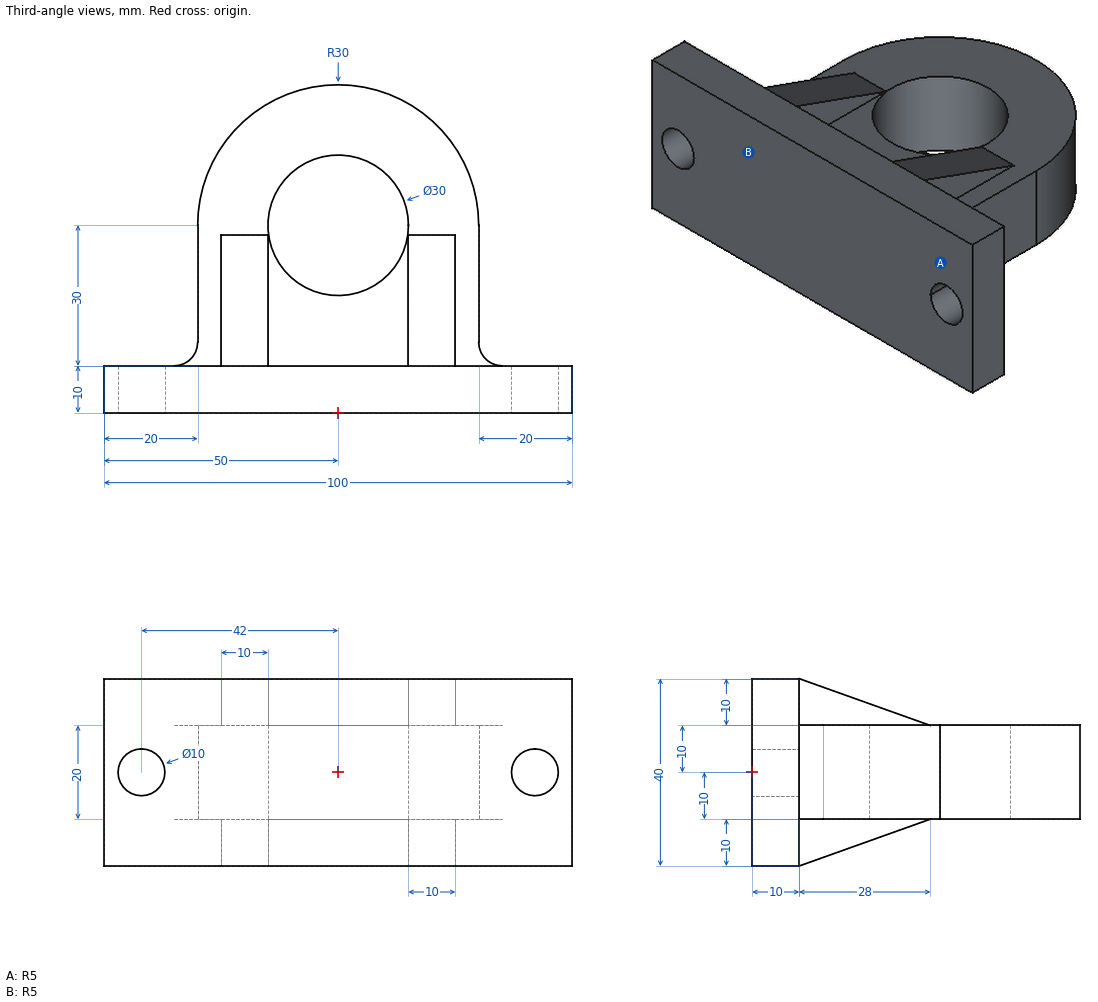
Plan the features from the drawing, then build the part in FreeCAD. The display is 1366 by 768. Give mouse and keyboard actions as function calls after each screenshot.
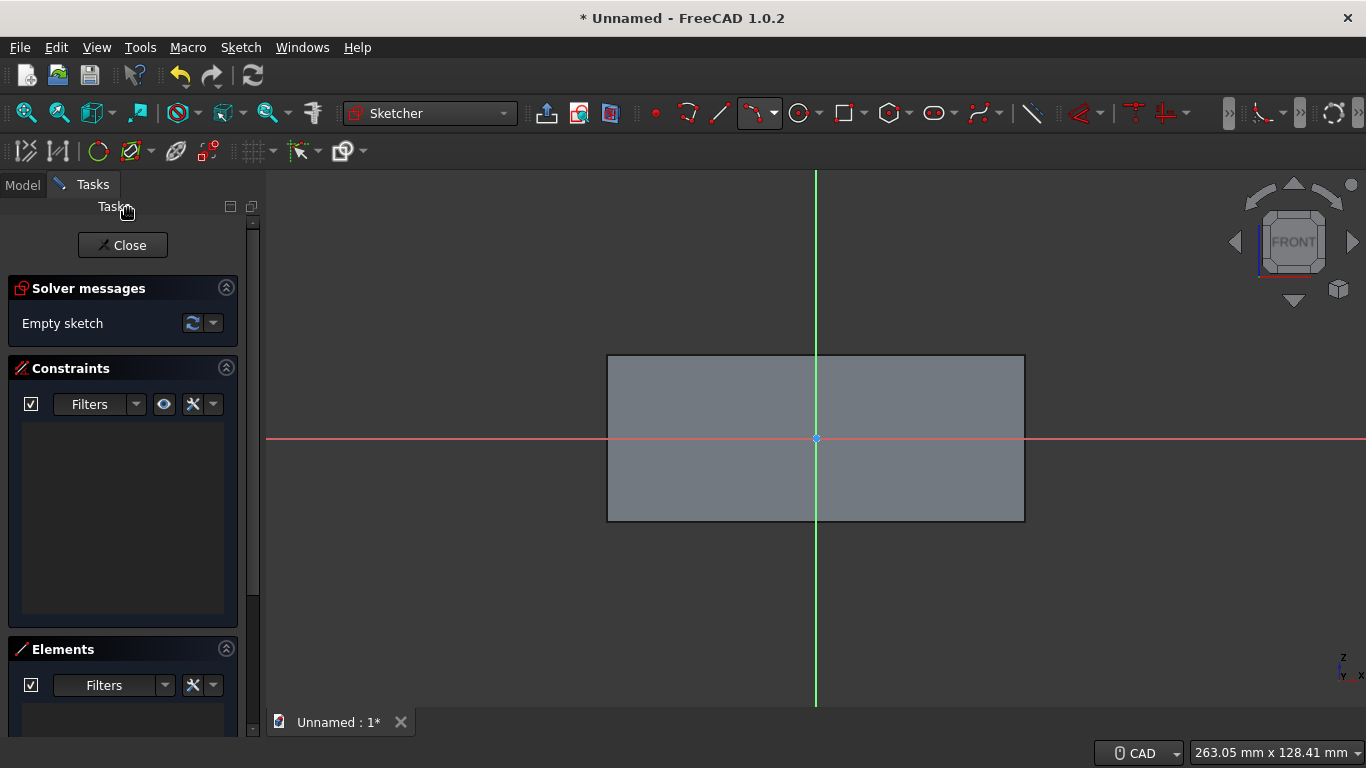
scroll(624, 438, up, 10)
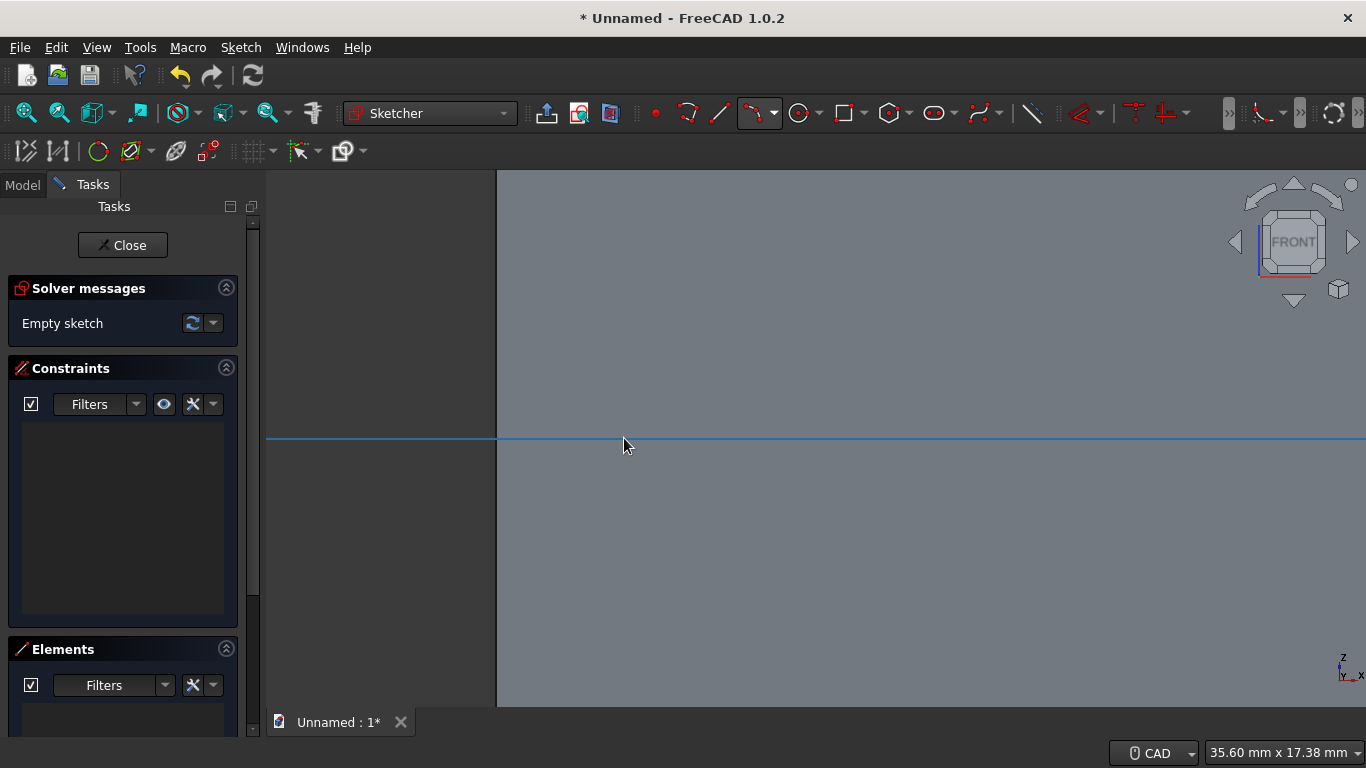
click(800, 114)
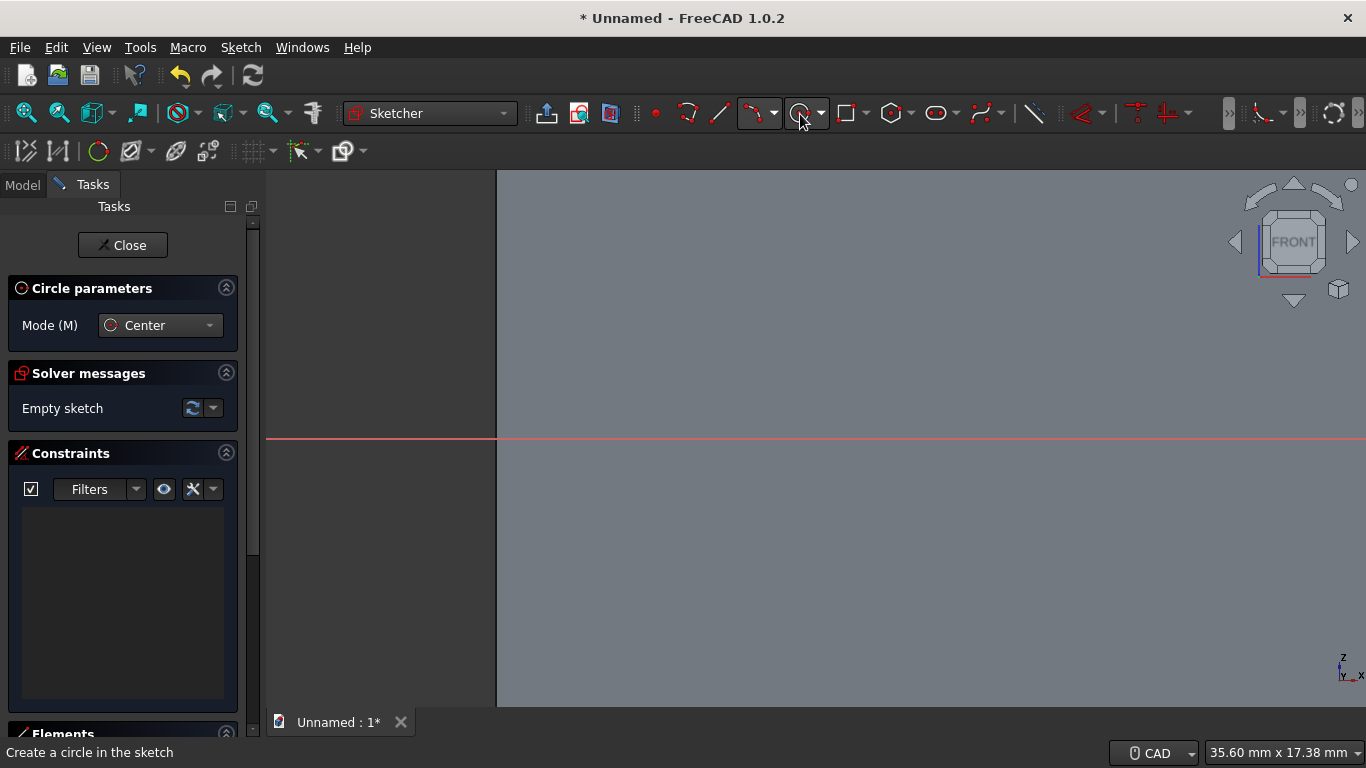
click(743, 438)
move(852, 329)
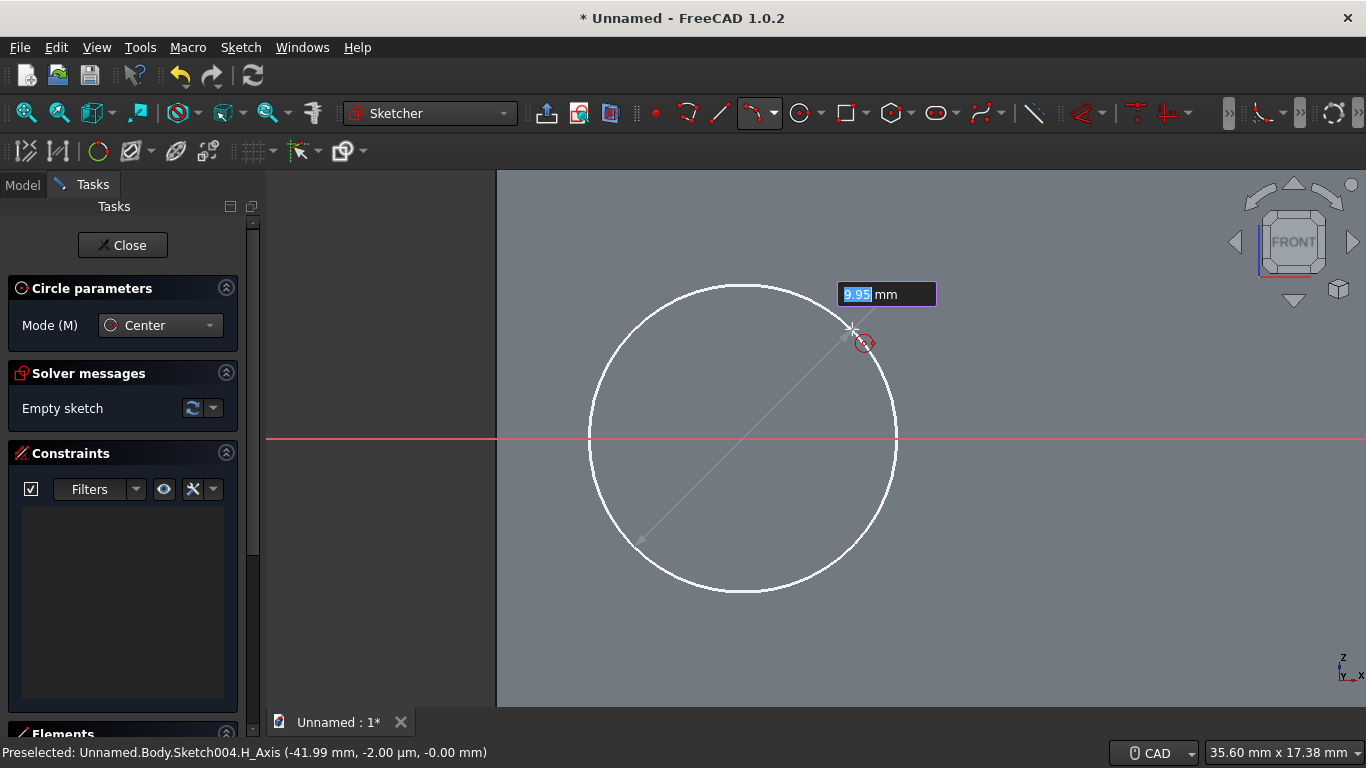
text(10)
key(Return)
key(Escape)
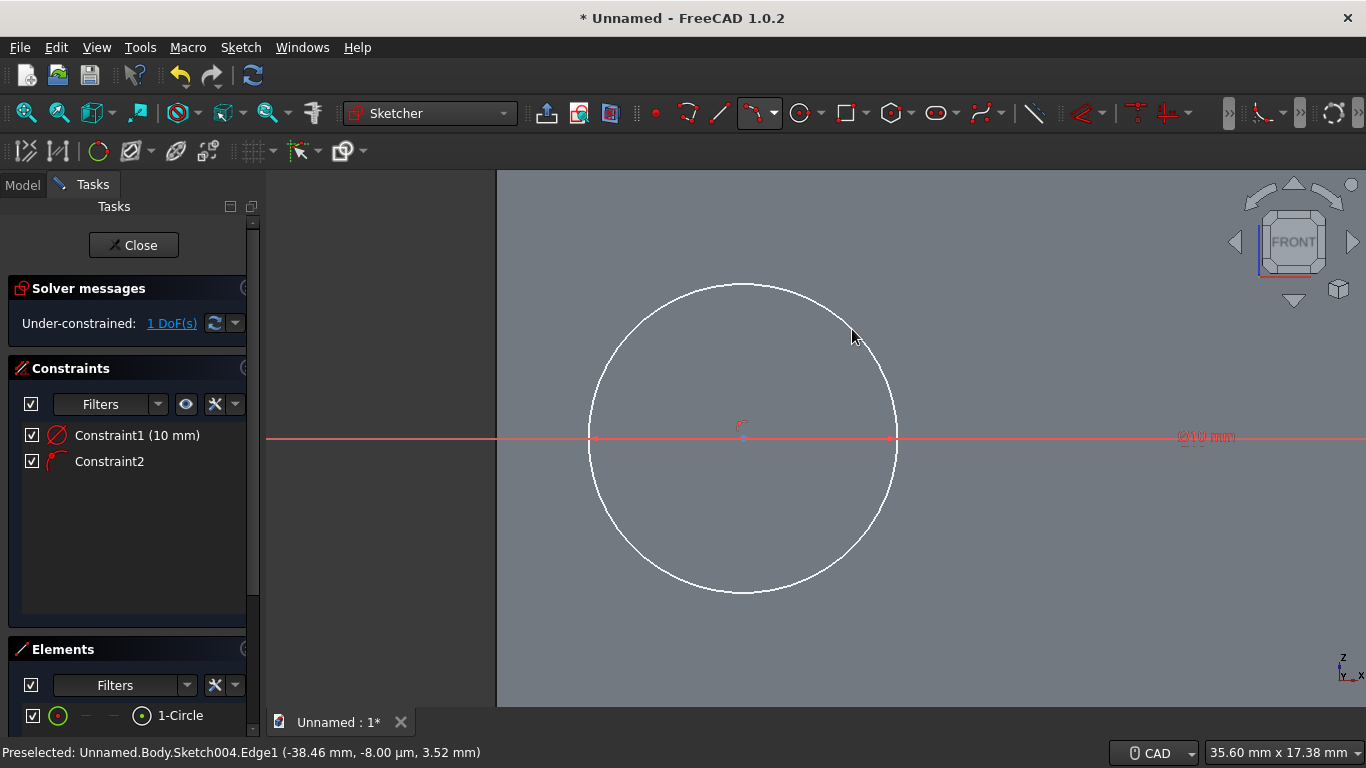
click(1082, 114)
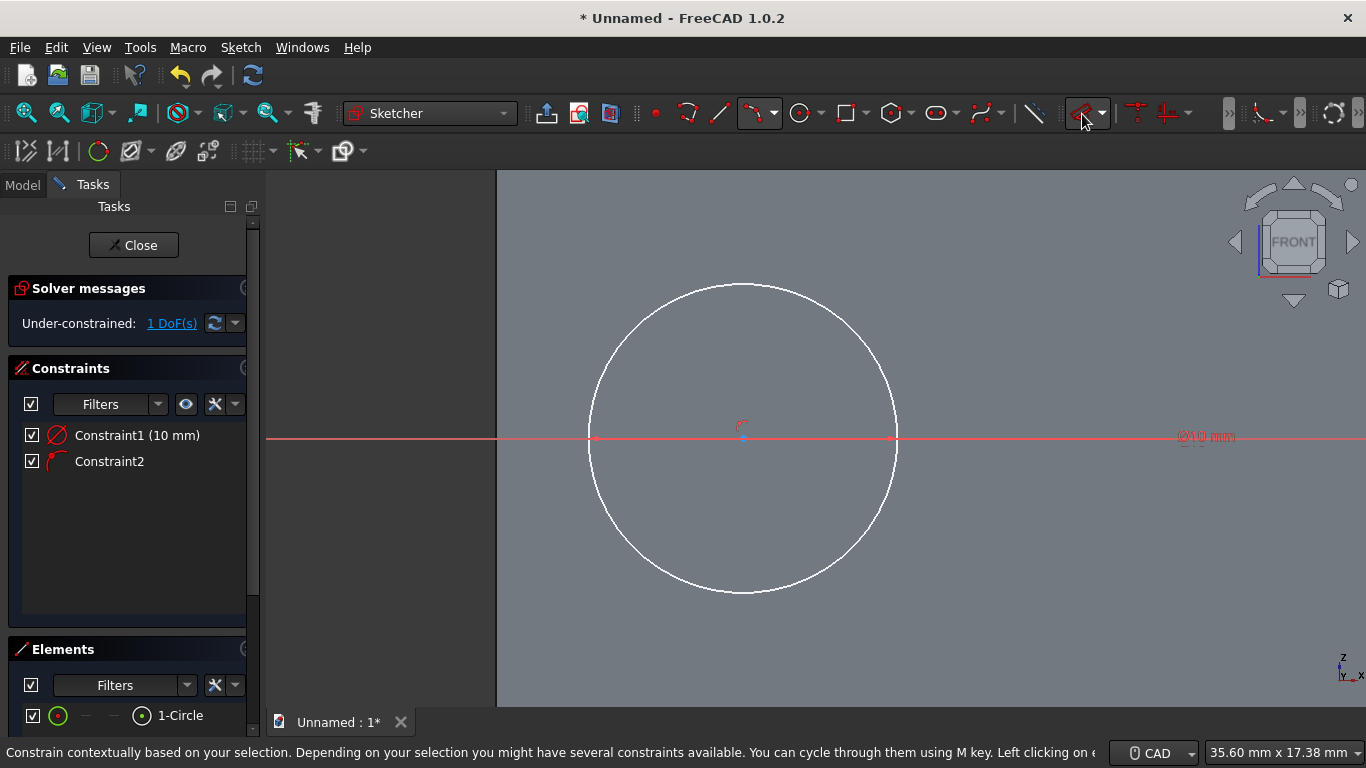
click(743, 438)
click(972, 472)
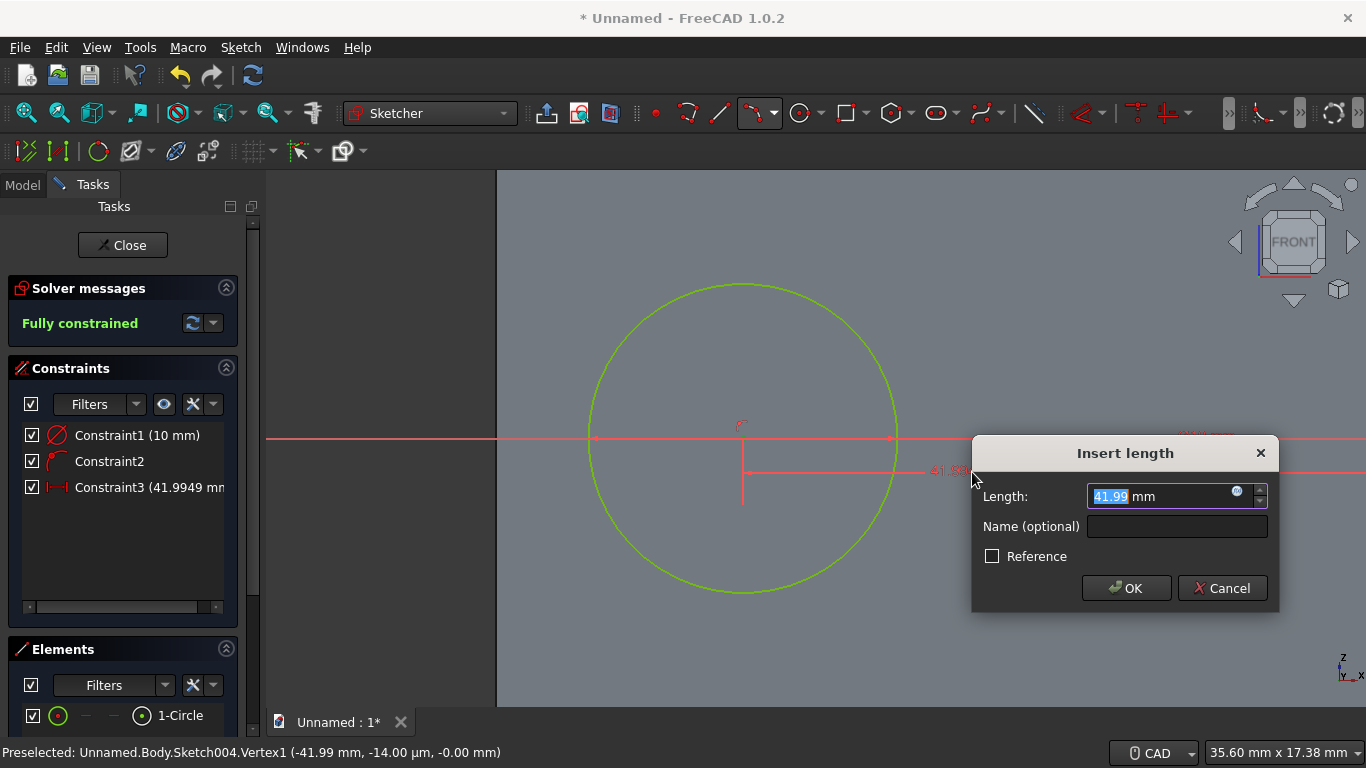
text(42)
key(Return)
key(Escape)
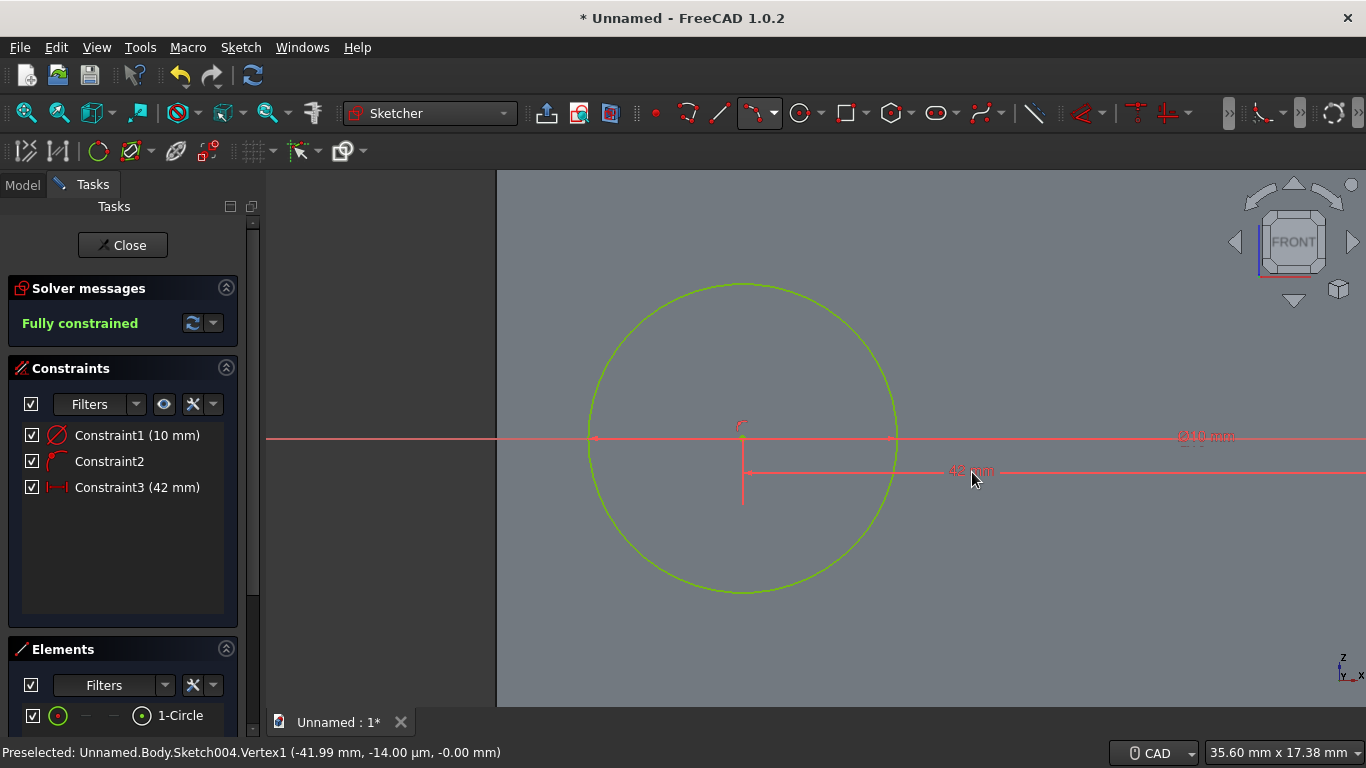
click(123, 245)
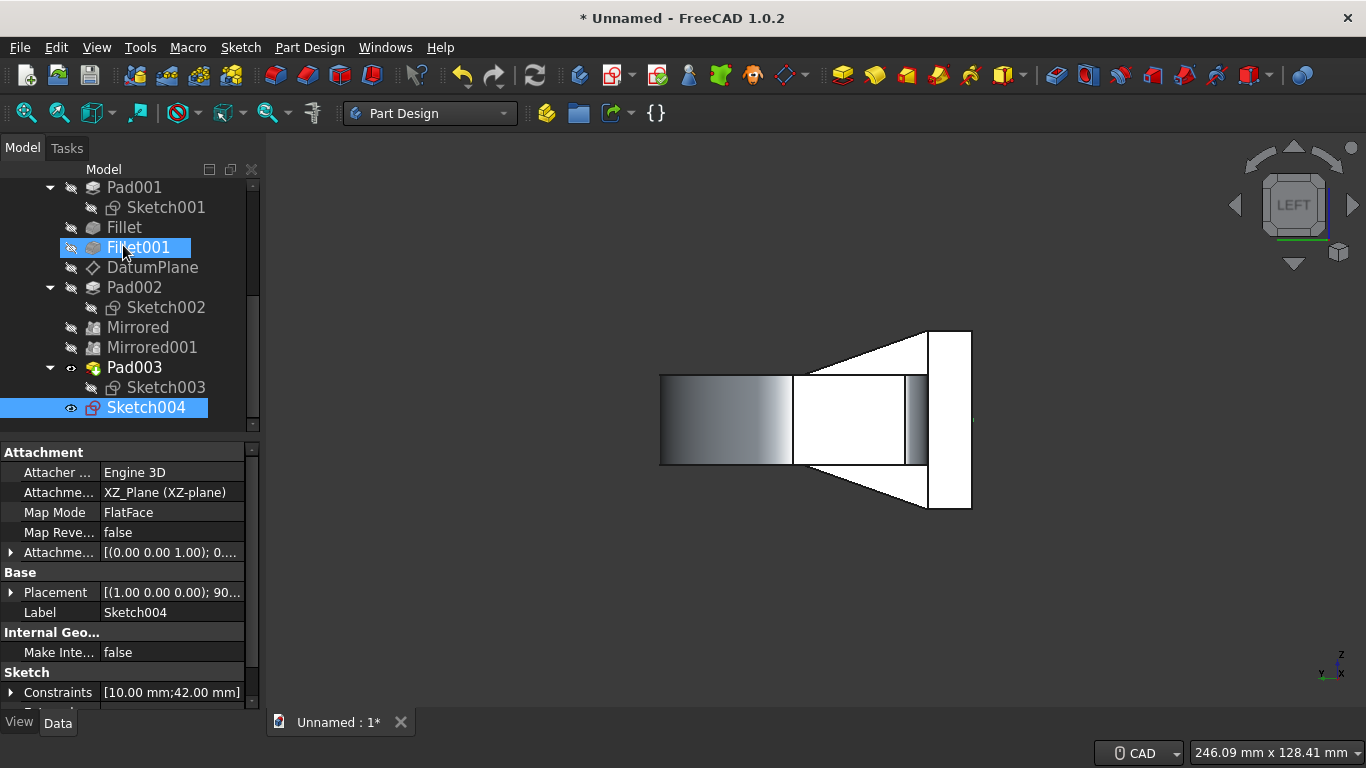
click(1058, 76)